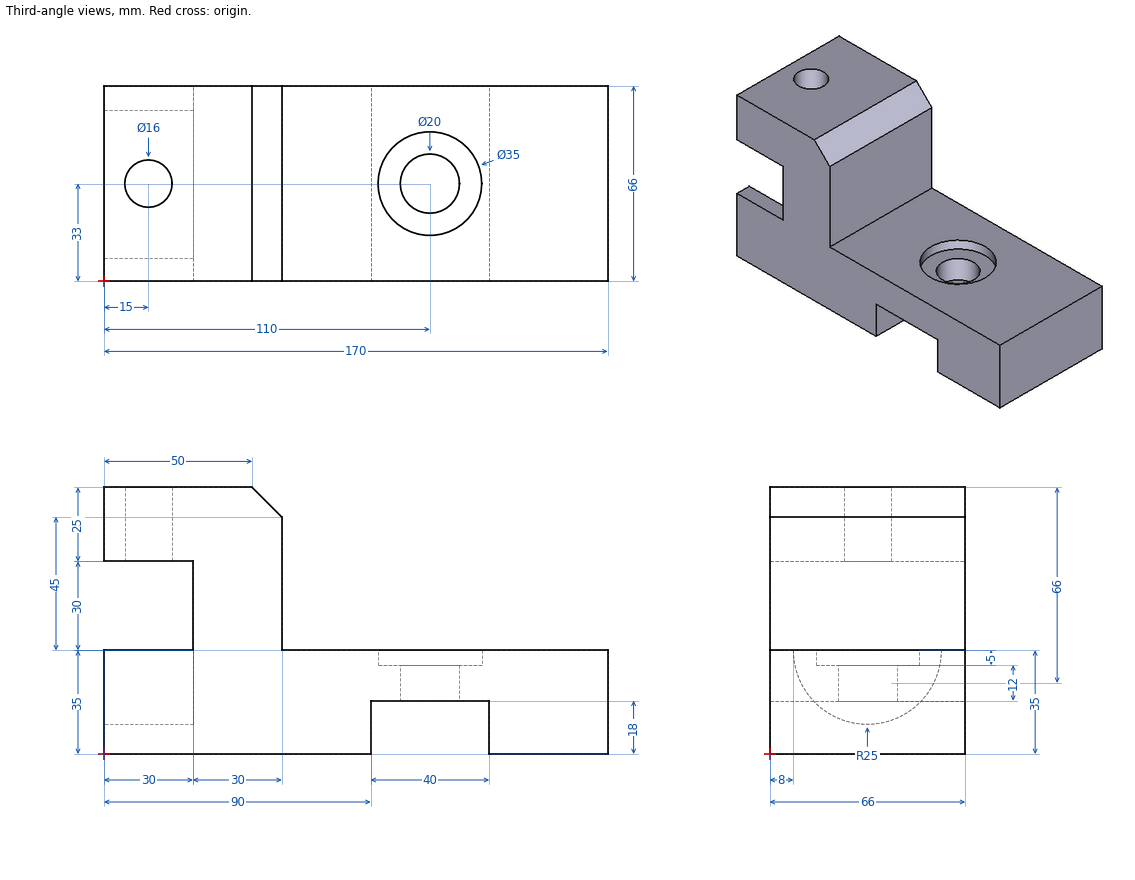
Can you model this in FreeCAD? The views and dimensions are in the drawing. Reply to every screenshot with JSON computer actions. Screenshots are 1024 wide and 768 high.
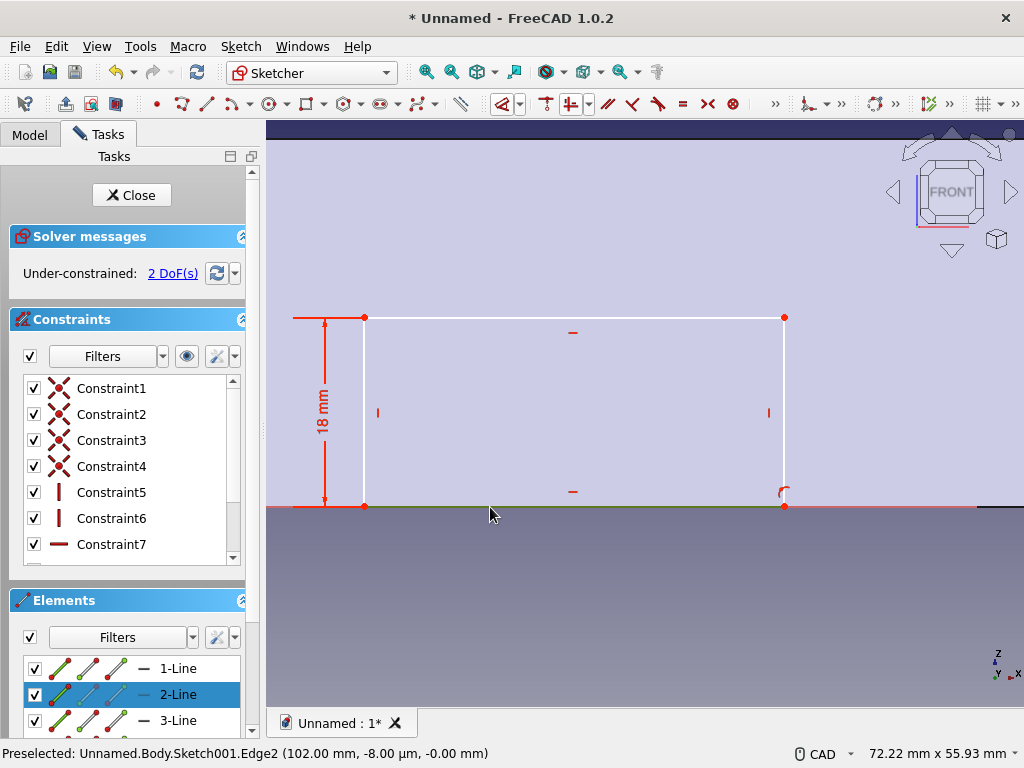
{"action": "key", "text": "l"}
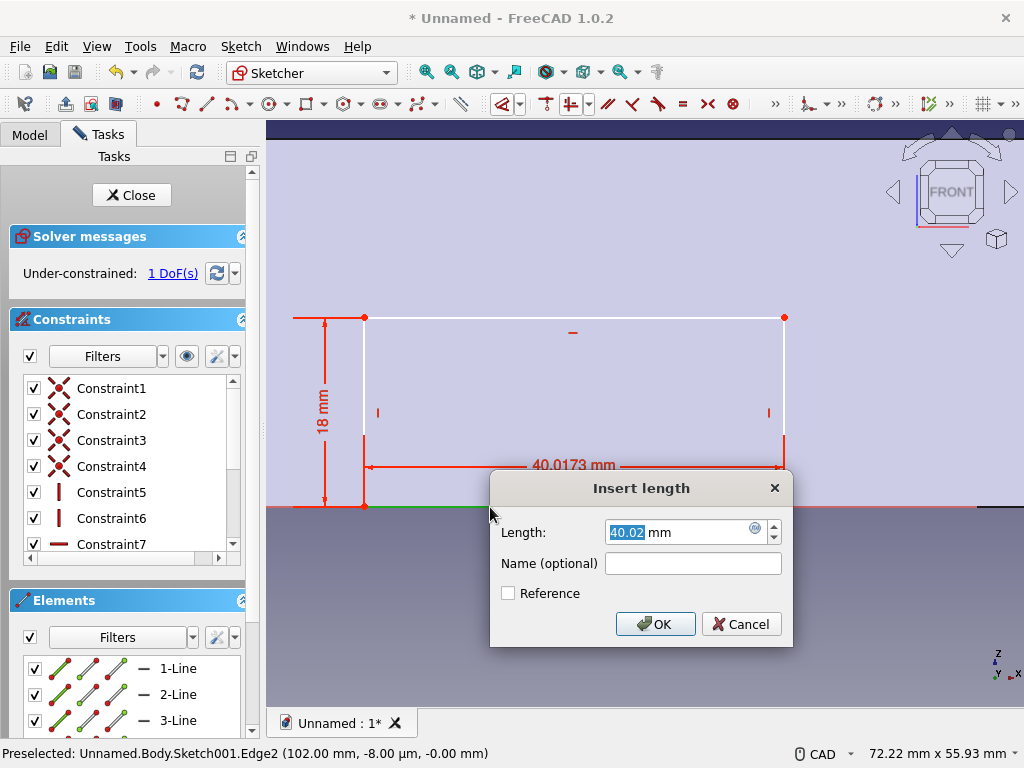
{"action": "type", "text": "40"}
{"action": "key", "text": "Return"}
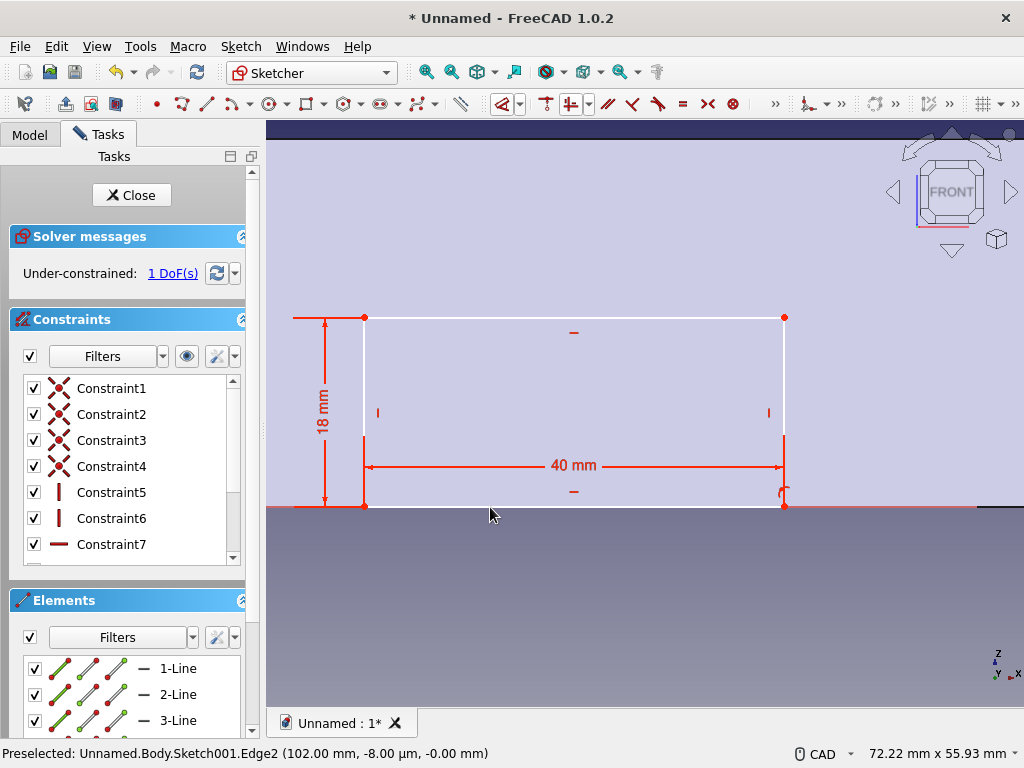
{"action": "left_click", "coordinate": [364, 318]}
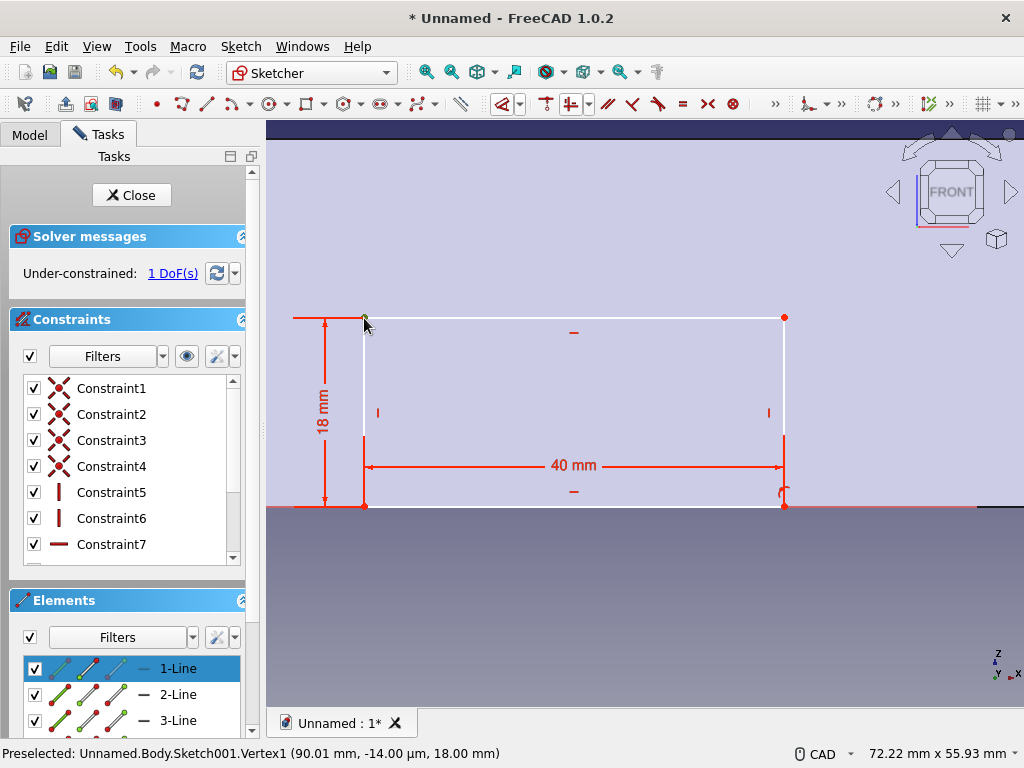
{"action": "key", "text": "l"}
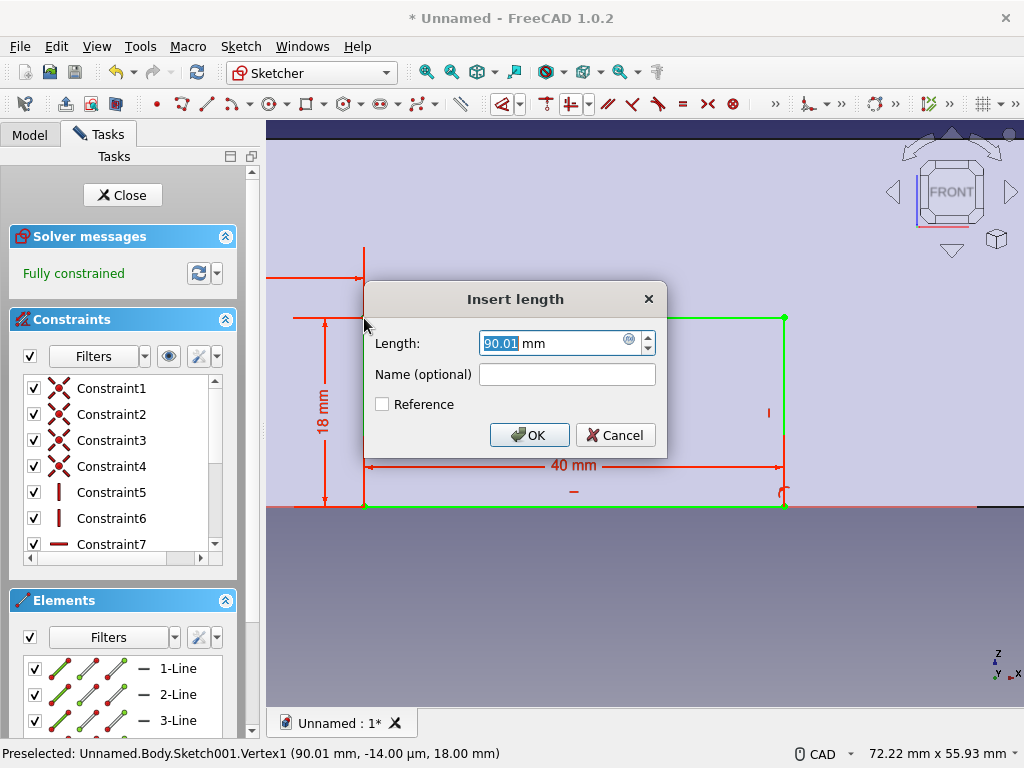
{"action": "type", "text": "90"}
{"action": "key", "text": "Return"}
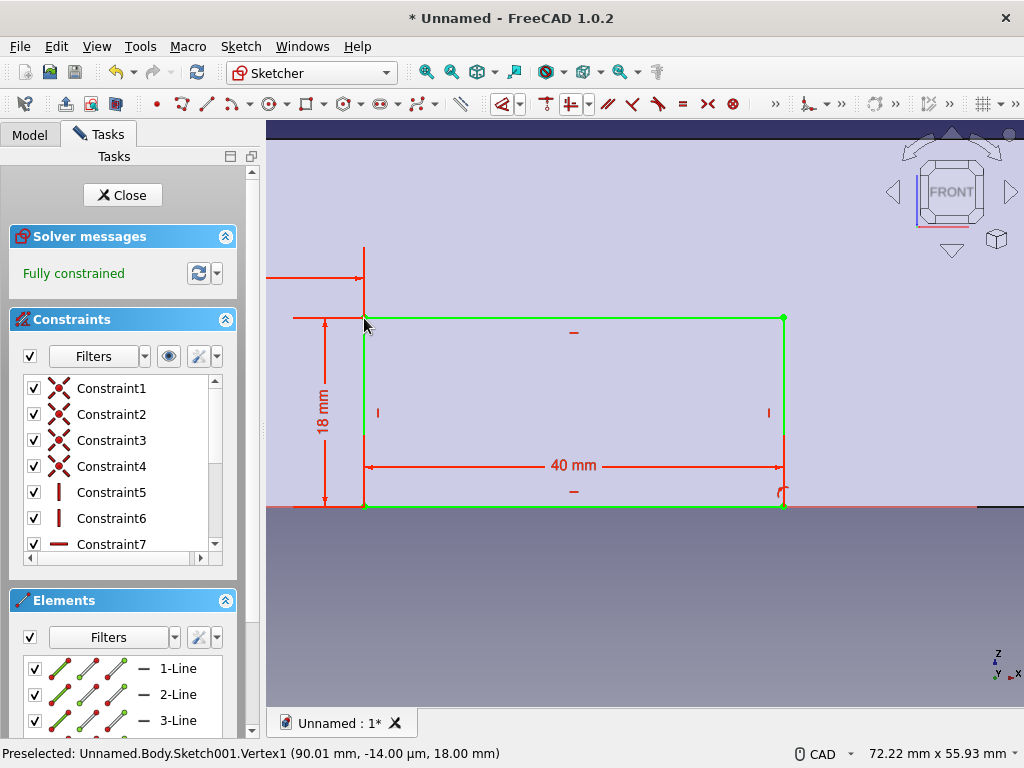
{"action": "left_click", "coordinate": [123, 195]}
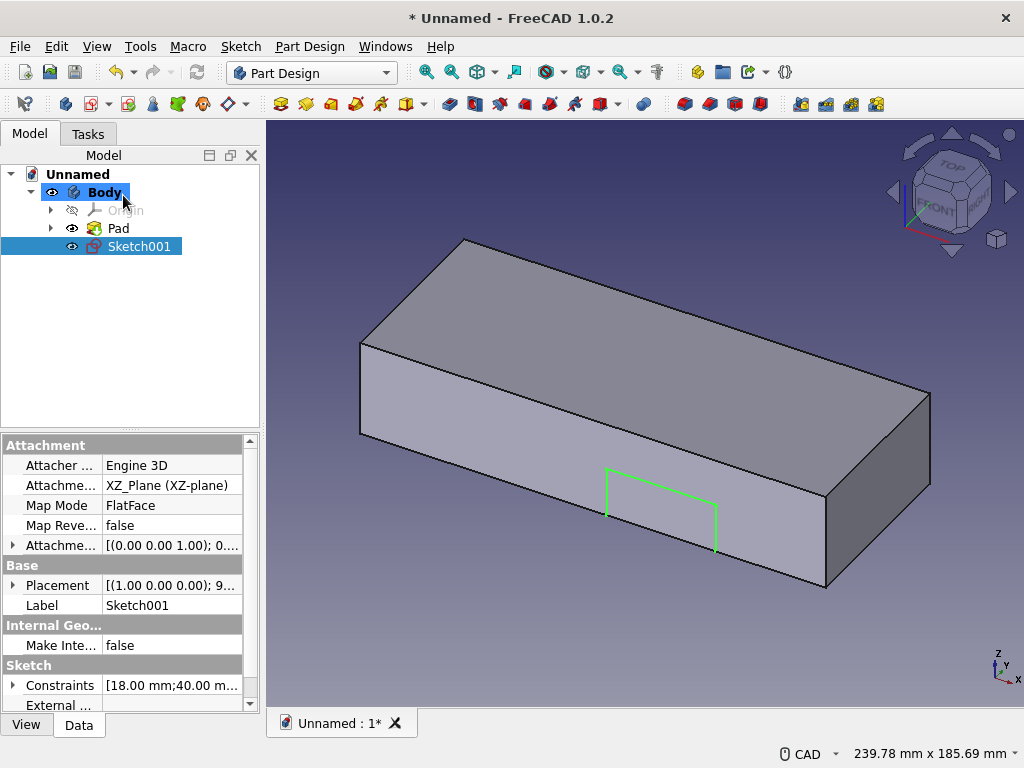
{"action": "left_click", "coordinate": [450, 104]}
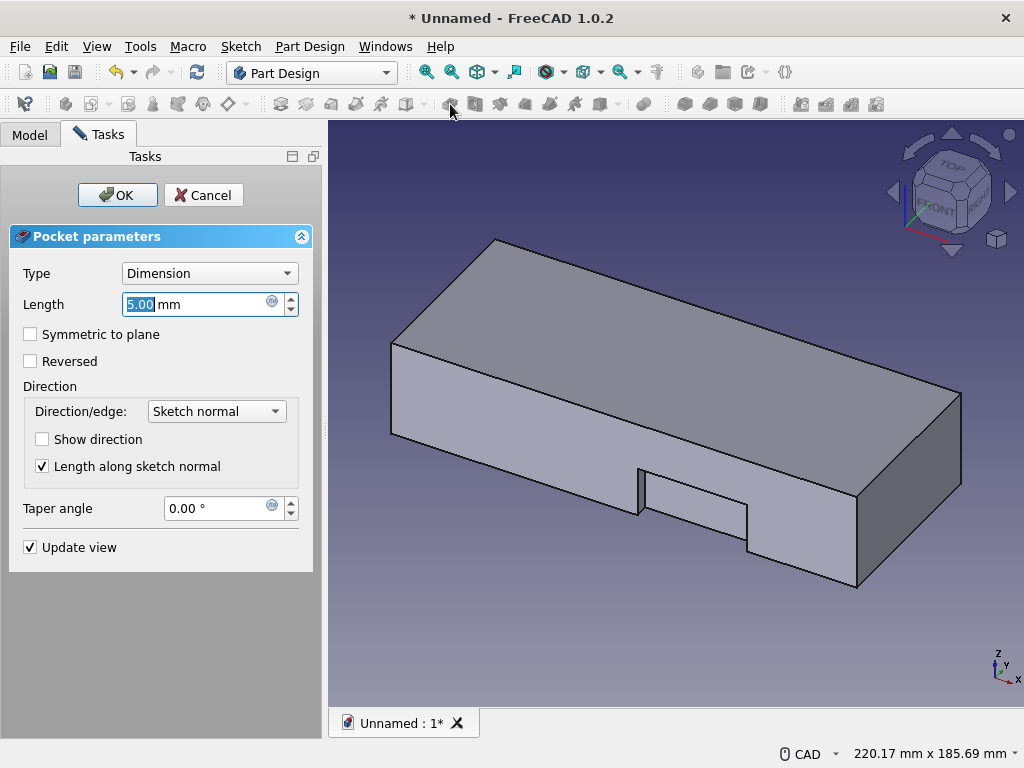
{"action": "type", "text": "66"}
{"action": "key", "text": "Tab"}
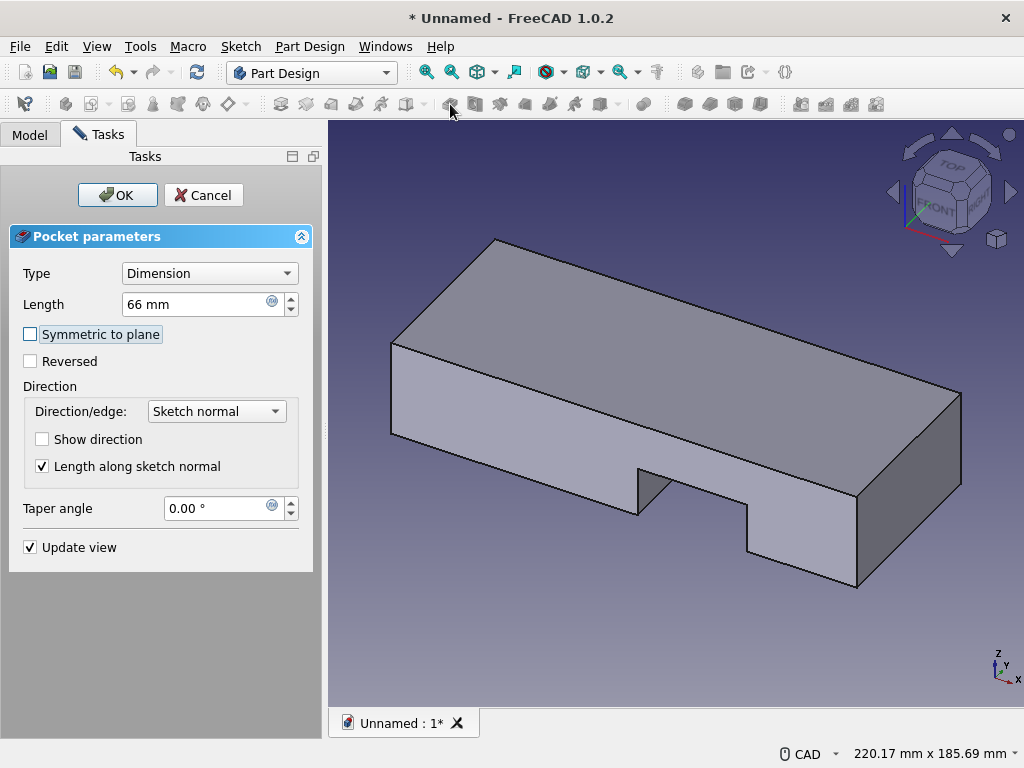
{"action": "left_click", "coordinate": [118, 195]}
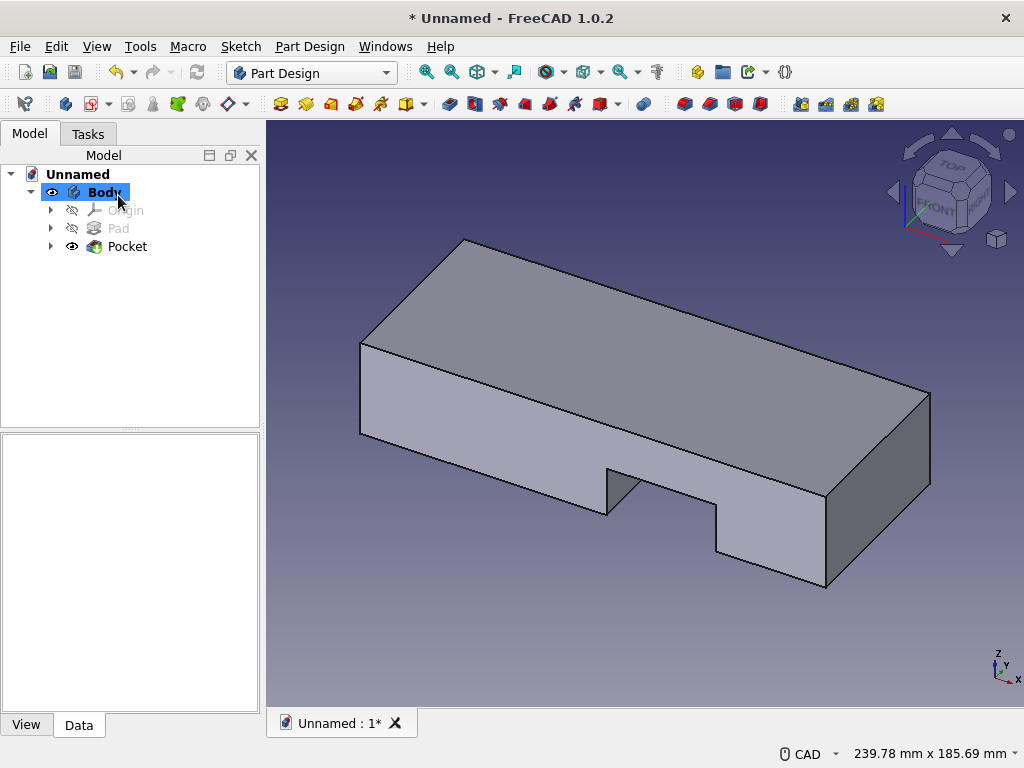
{"action": "left_click", "coordinate": [778, 411]}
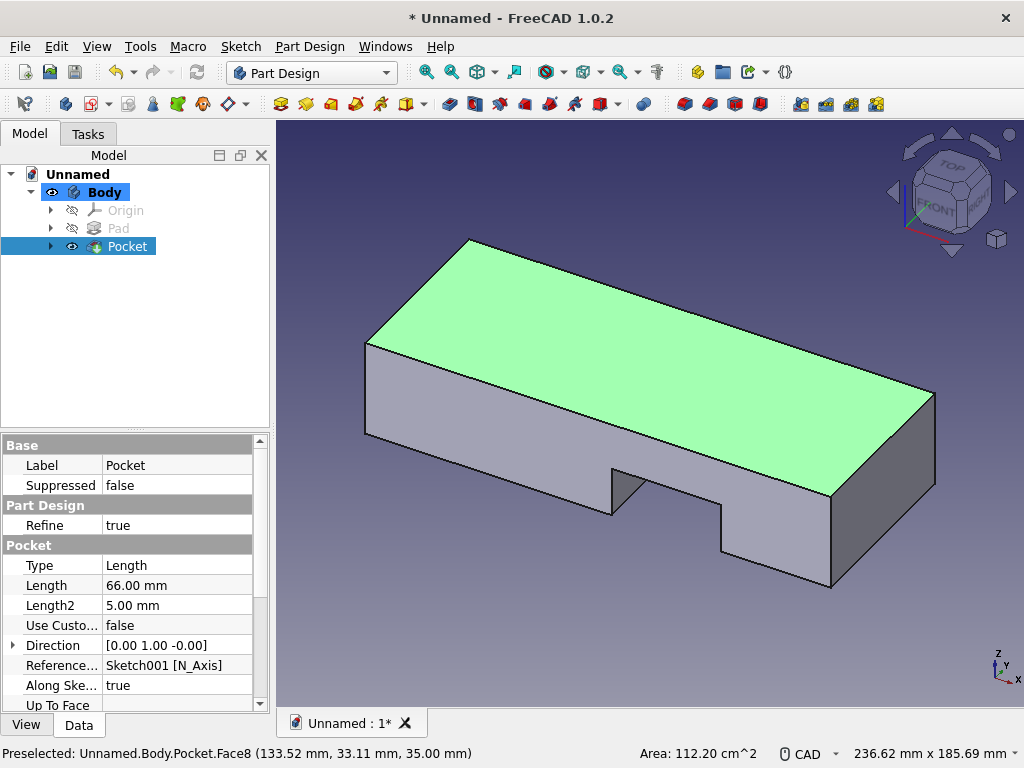
{"action": "left_click", "coordinate": [90, 104]}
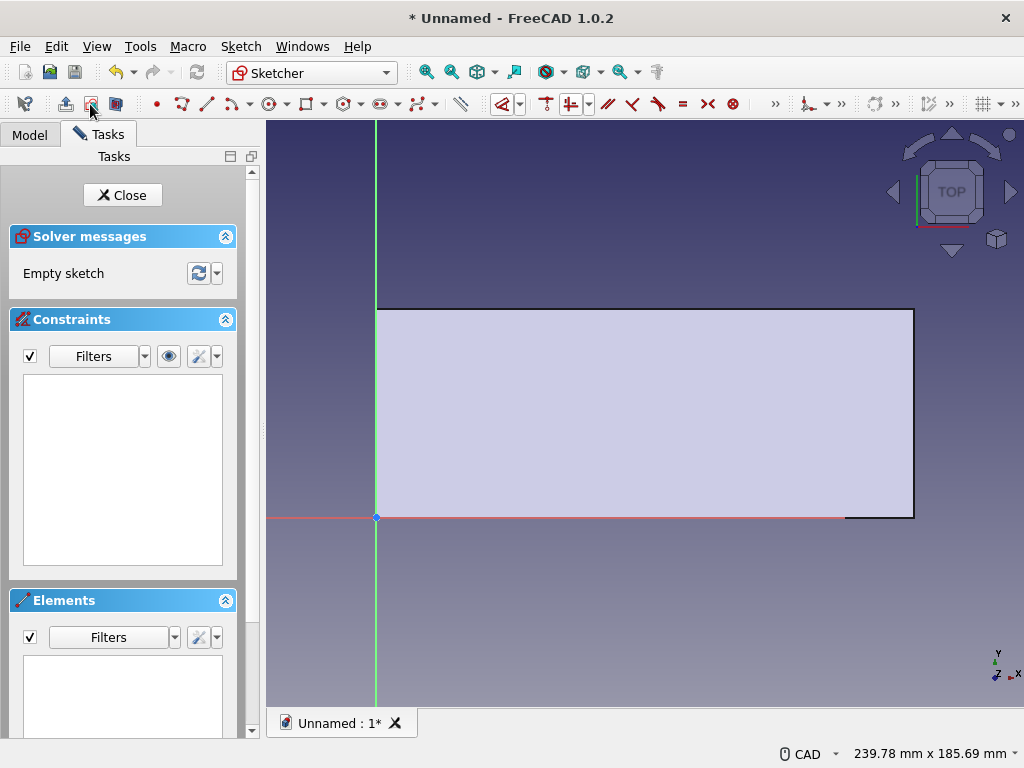
{"action": "scroll", "coordinate": [788, 414], "scroll_direction": "up", "scroll_amount": 6}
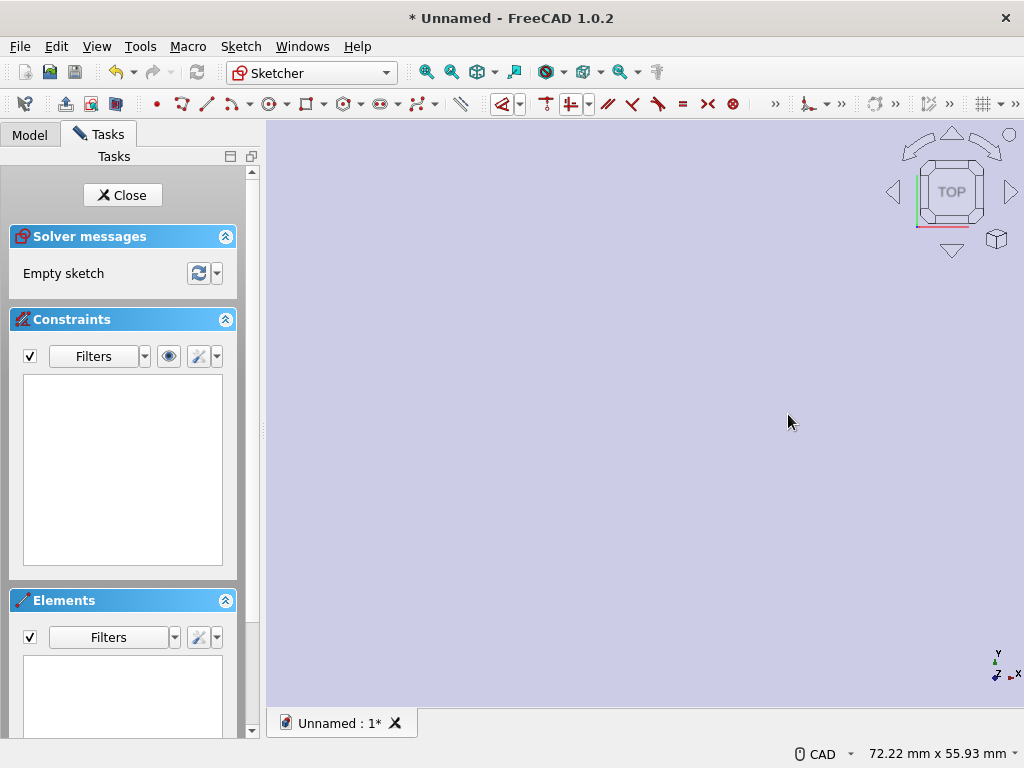
{"action": "left_click", "coordinate": [268, 104]}